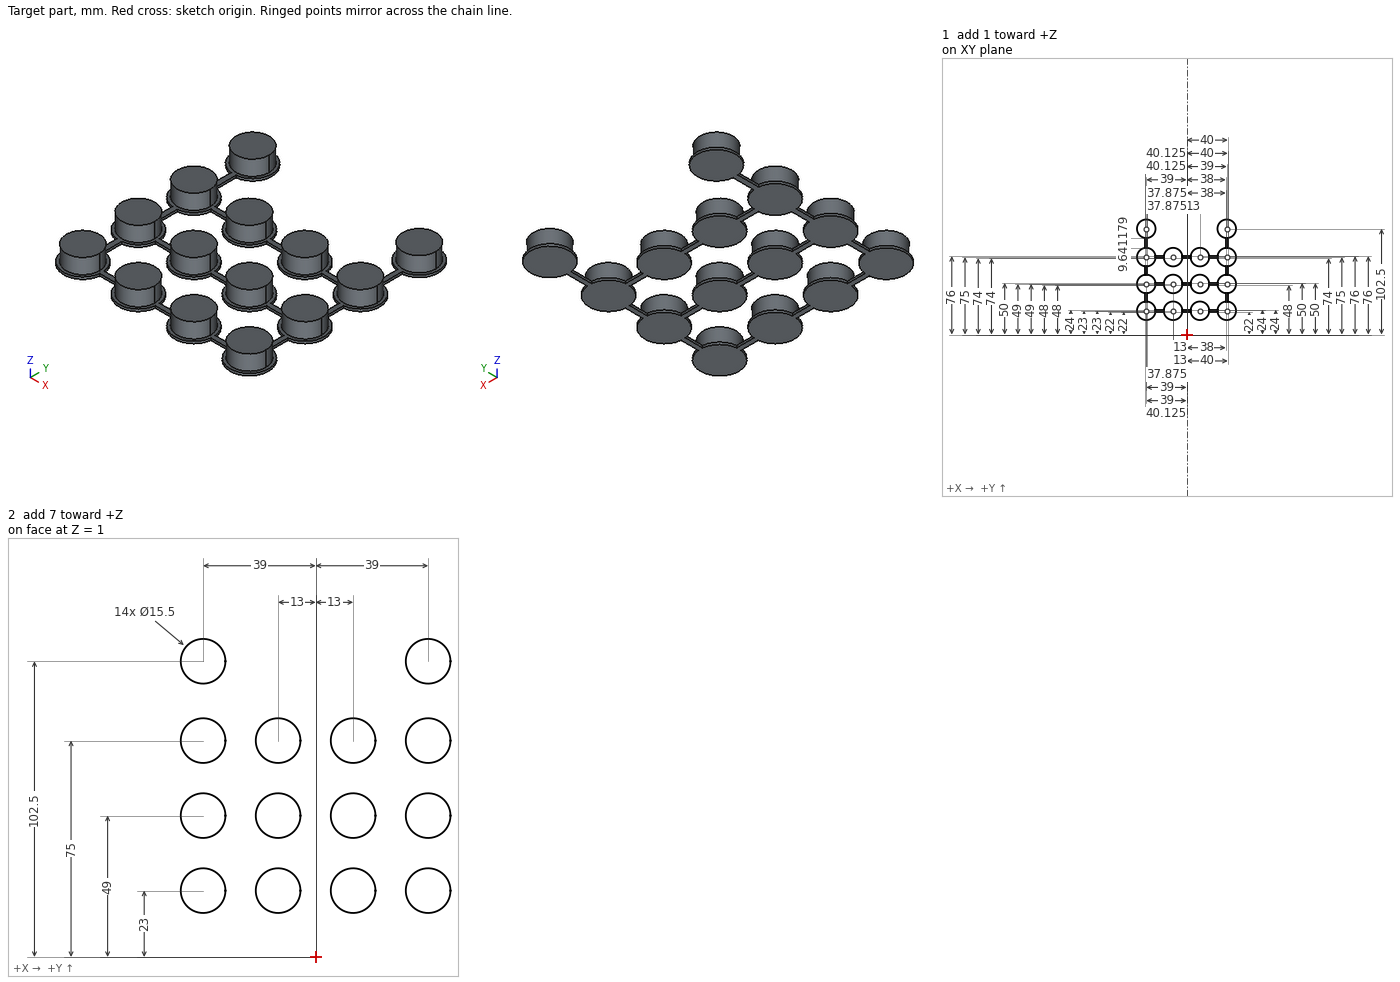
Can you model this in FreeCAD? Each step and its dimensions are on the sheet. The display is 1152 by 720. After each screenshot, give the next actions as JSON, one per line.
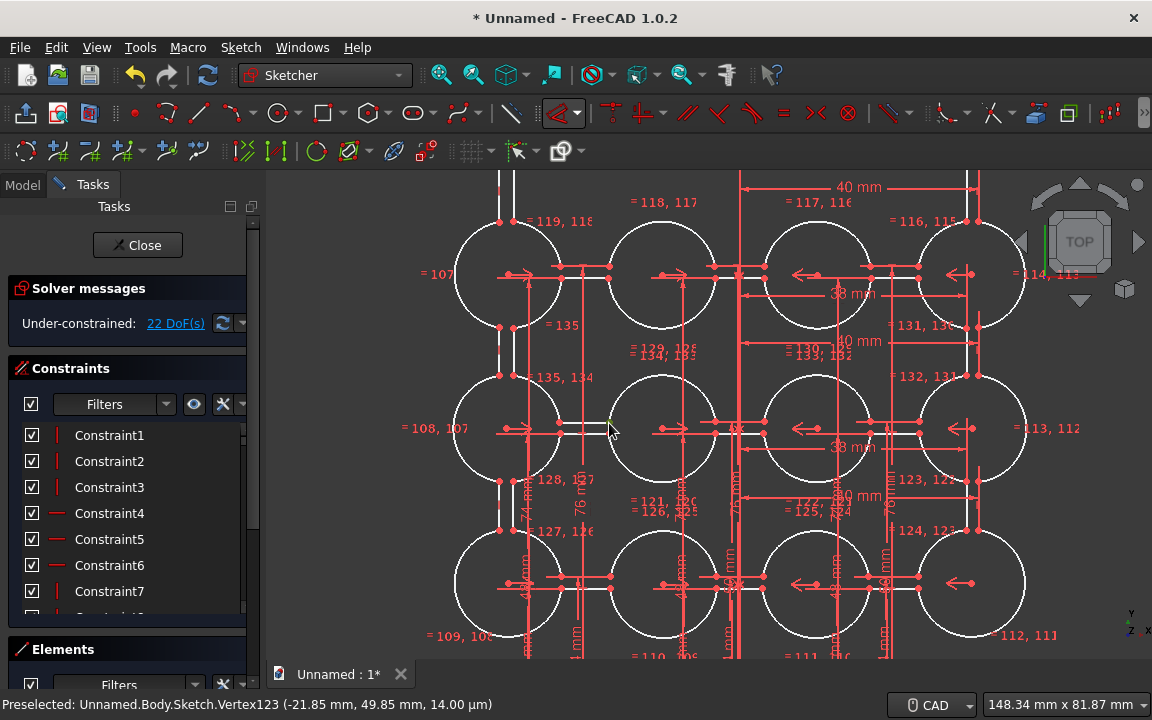
{"action": "left_click", "coordinate": [580, 114]}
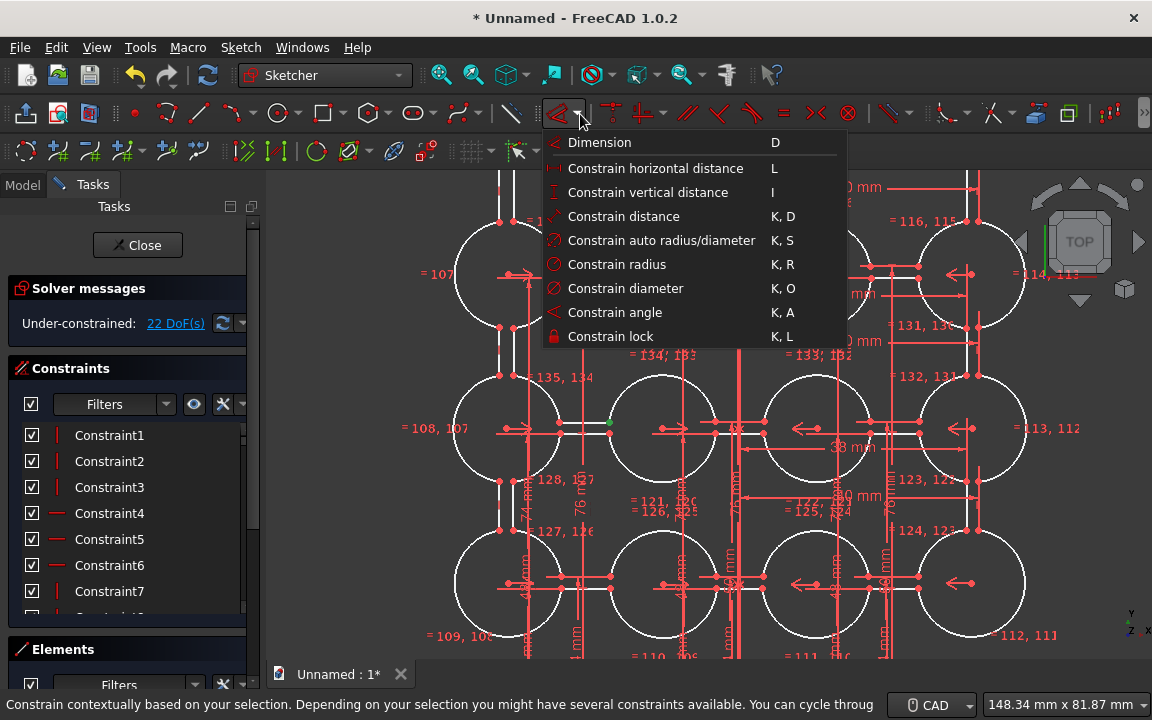
{"action": "left_click", "coordinate": [695, 192]}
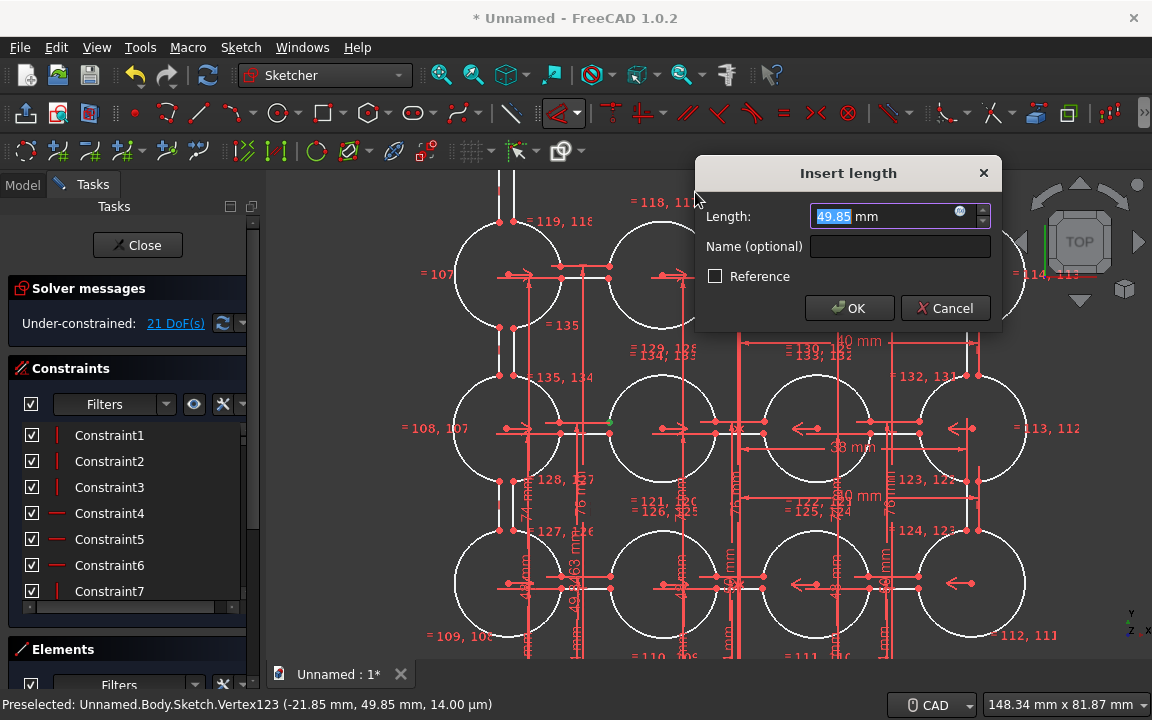
{"action": "type", "text": "50"}
{"action": "key", "text": "Return"}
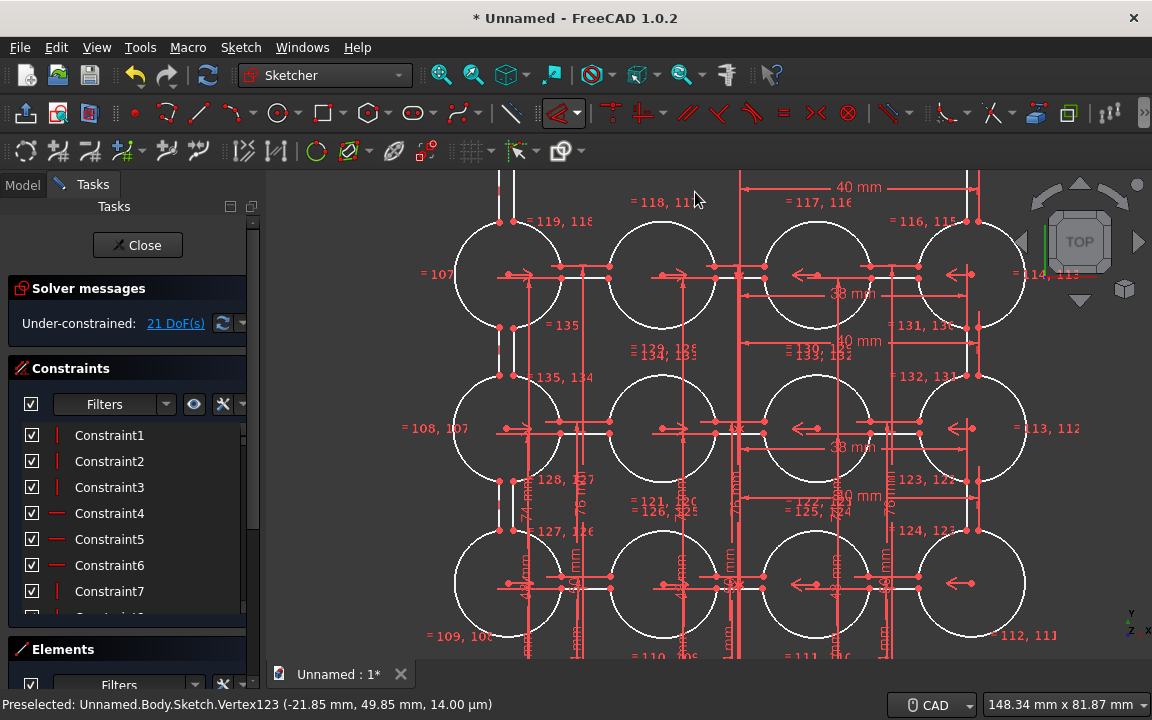
{"action": "left_click", "coordinate": [508, 275]}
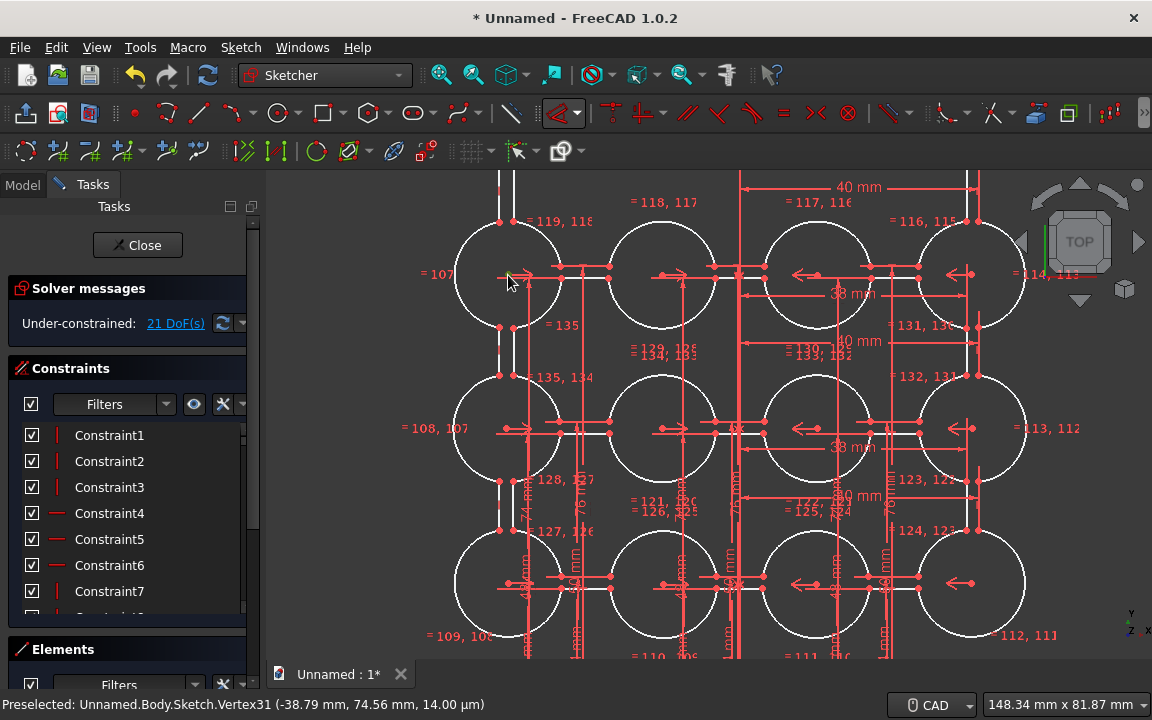
{"action": "left_click", "coordinate": [580, 114]}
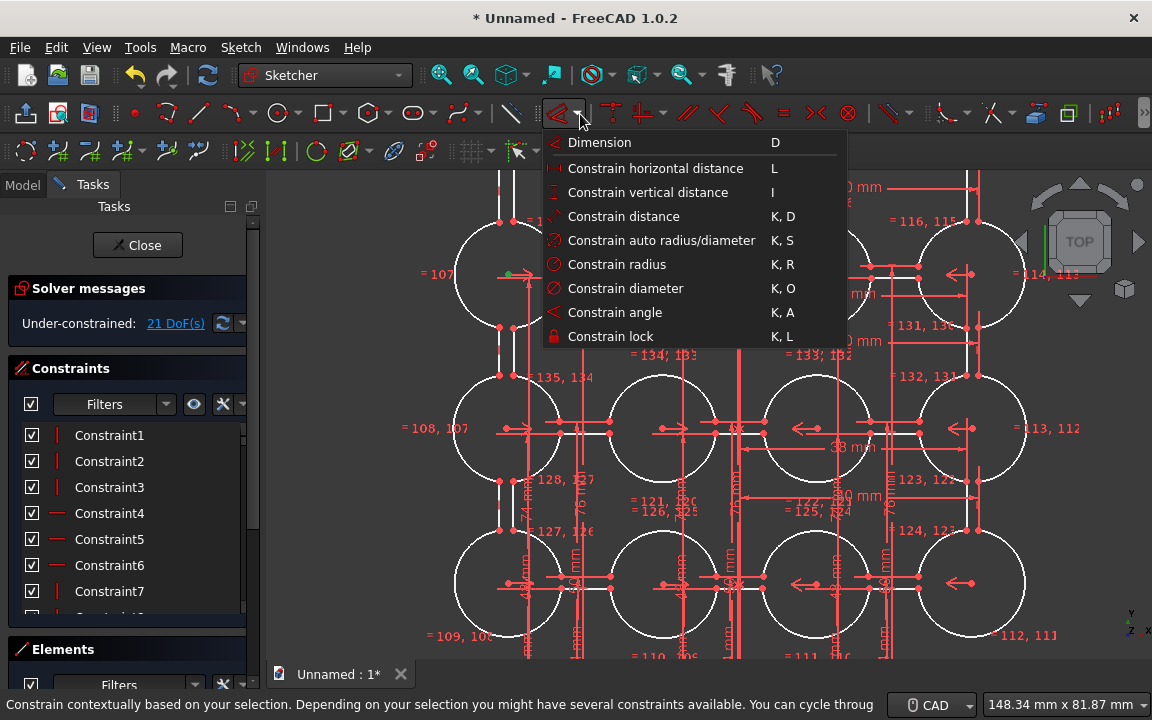
{"action": "left_click", "coordinate": [695, 168]}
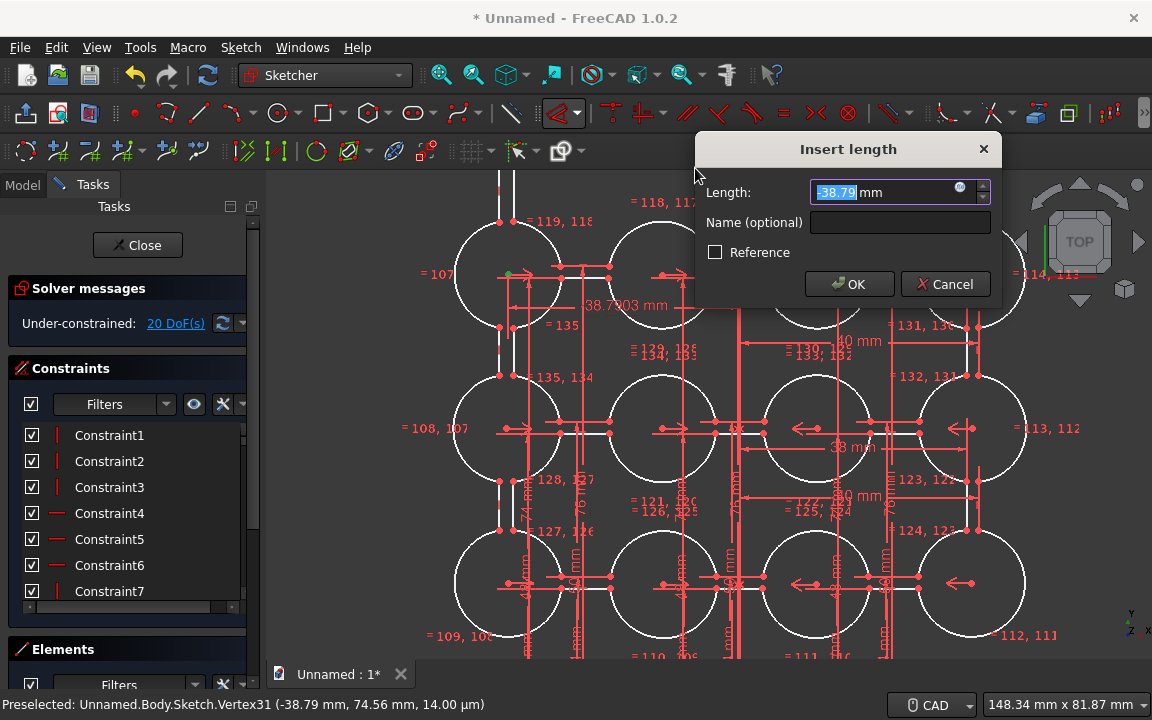
{"action": "type", "text": "-39"}
{"action": "key", "text": "Return"}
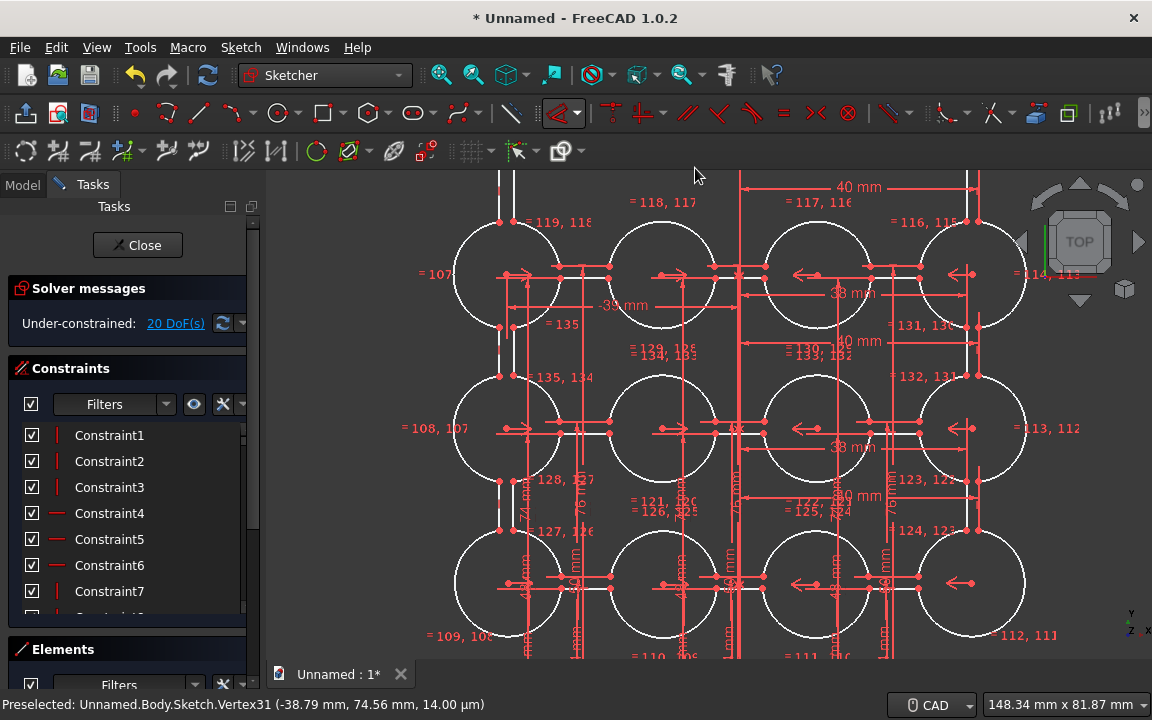
{"action": "left_click", "coordinate": [507, 275]}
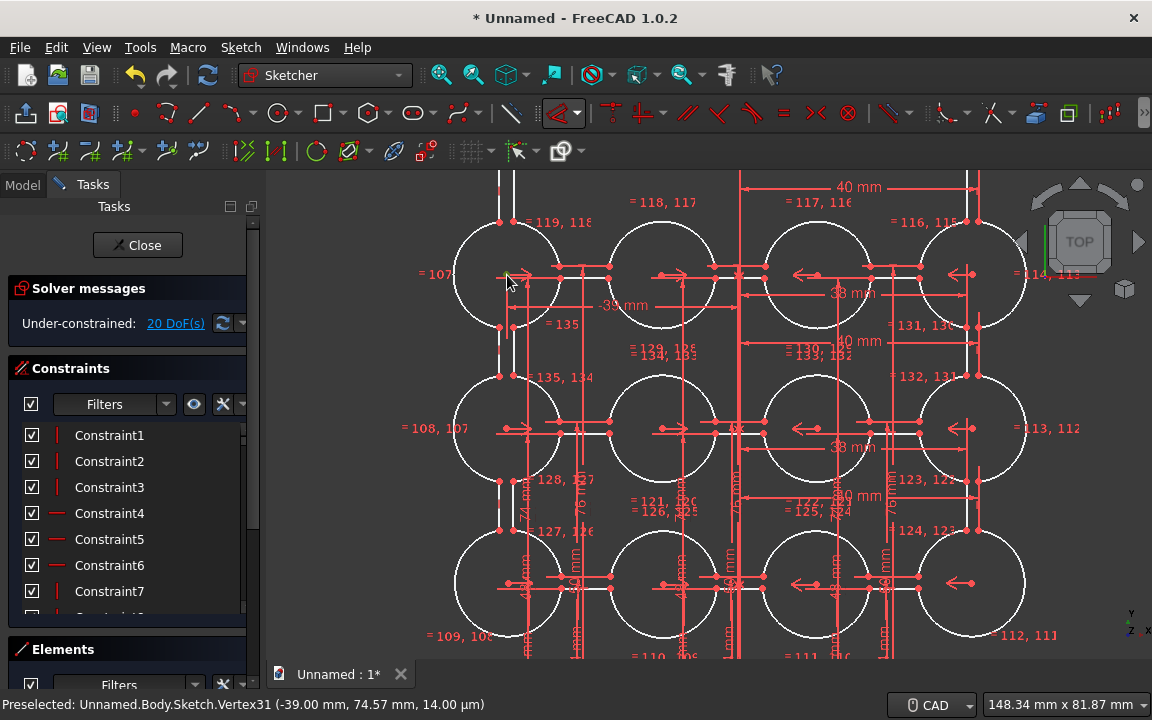
{"action": "left_click", "coordinate": [580, 114]}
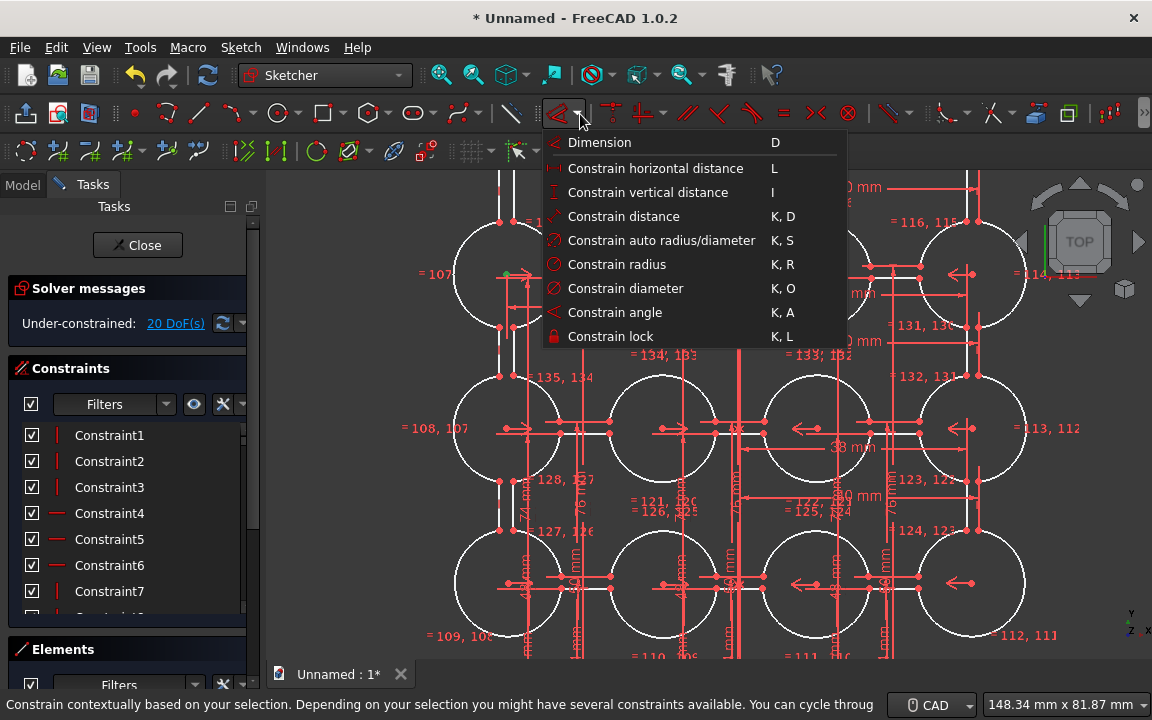
{"action": "left_click", "coordinate": [695, 192]}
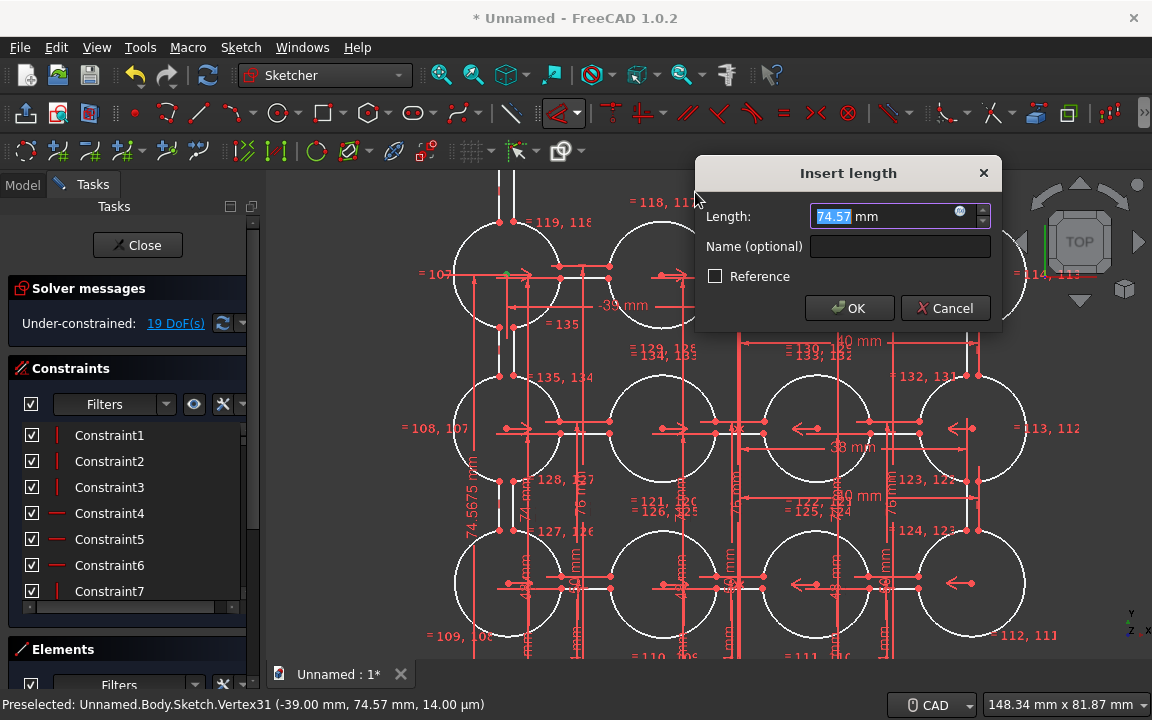
{"action": "type", "text": "75"}
{"action": "key", "text": "Return"}